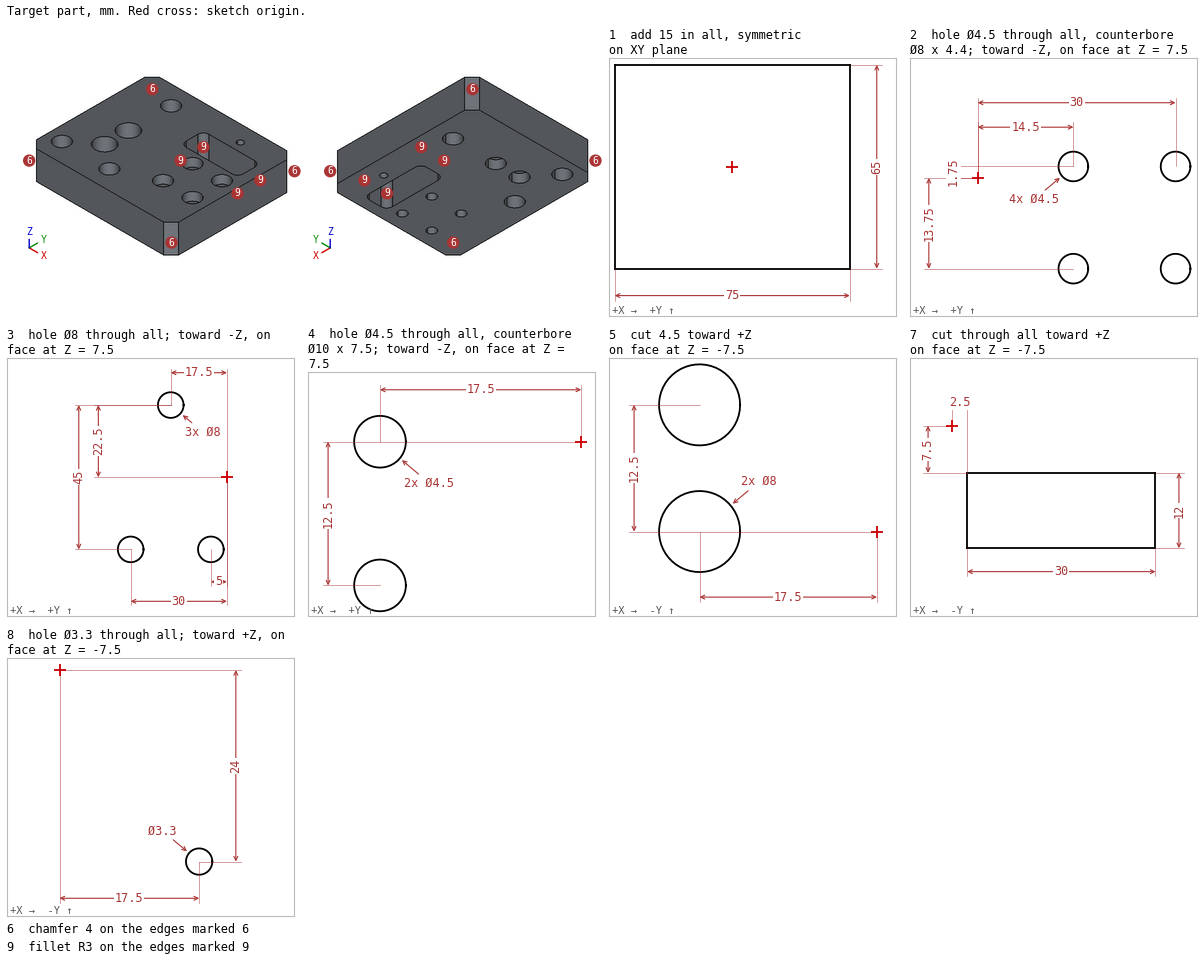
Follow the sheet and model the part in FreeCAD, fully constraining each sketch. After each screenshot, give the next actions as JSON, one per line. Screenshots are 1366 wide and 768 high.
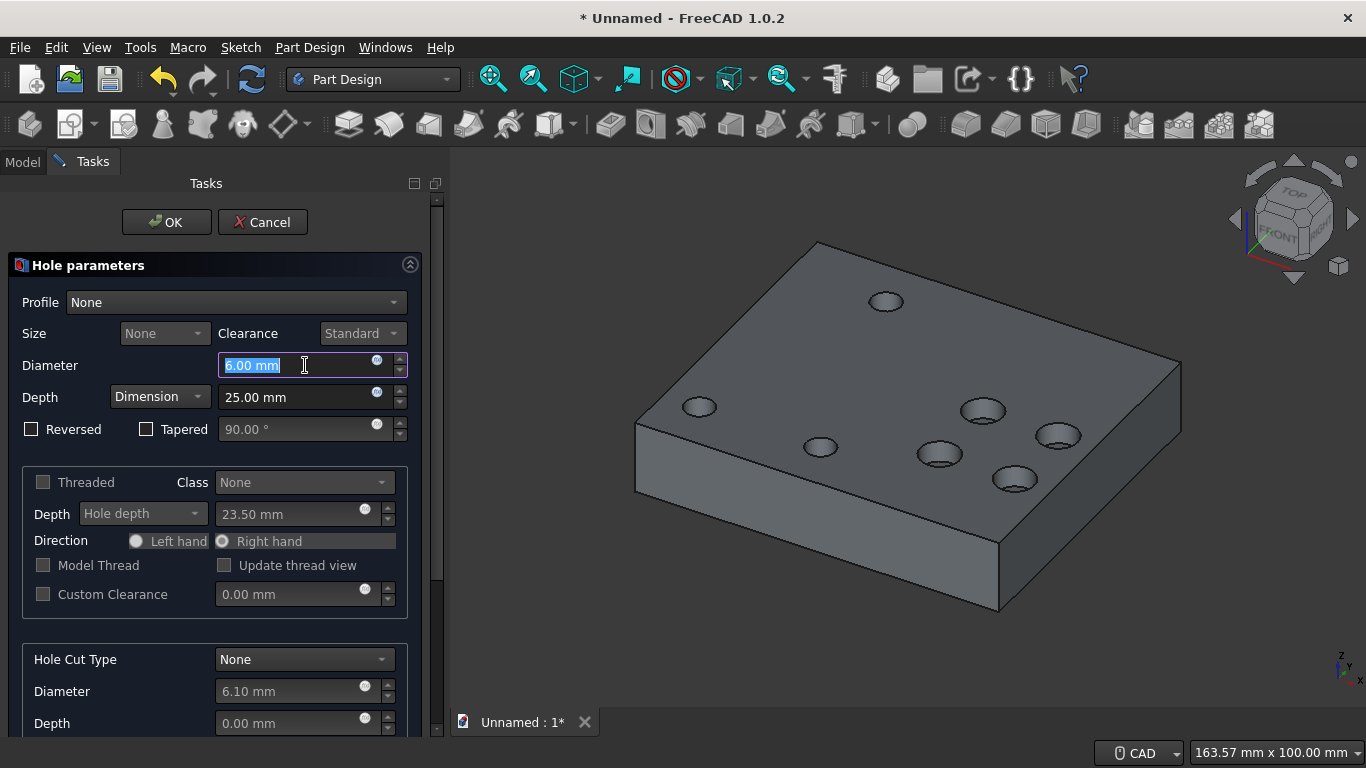
{"action": "type", "text": "8"}
{"action": "key", "text": "Tab"}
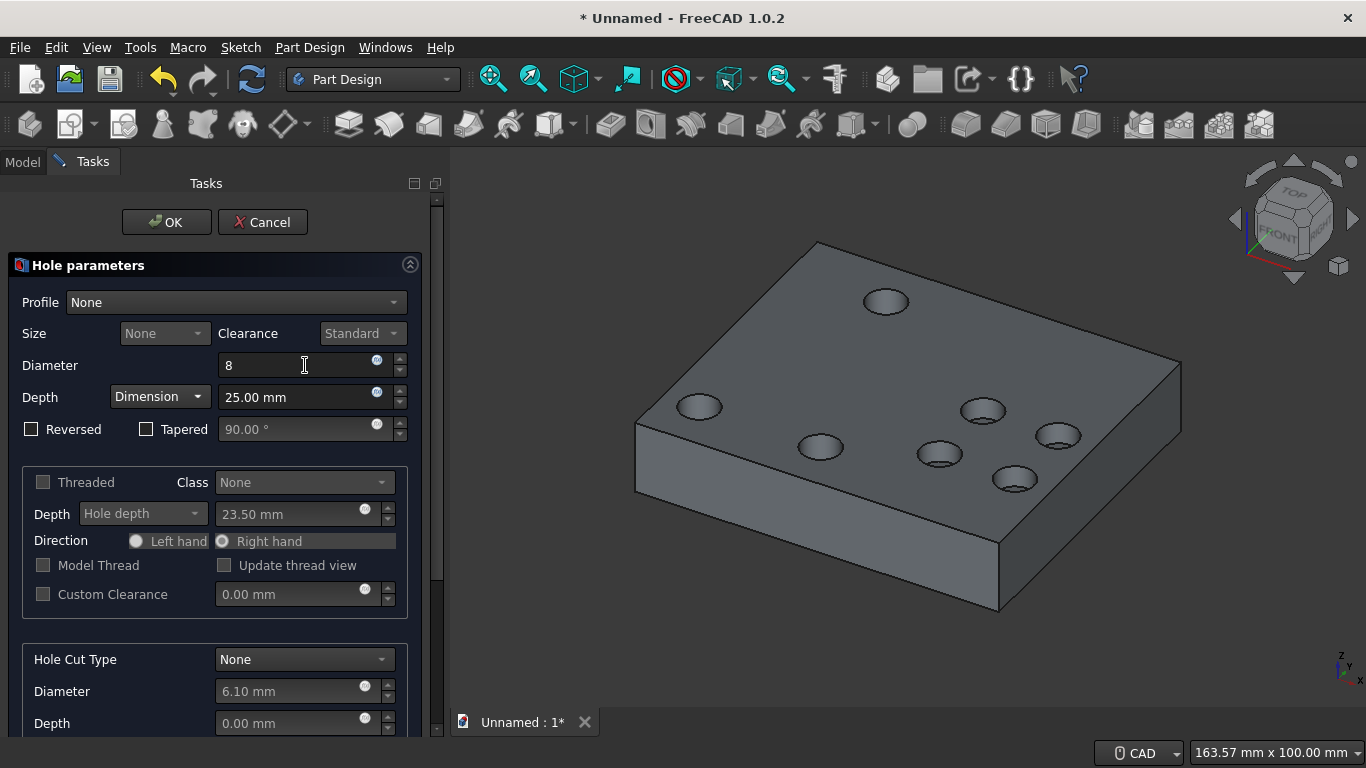
{"action": "left_click", "coordinate": [161, 396]}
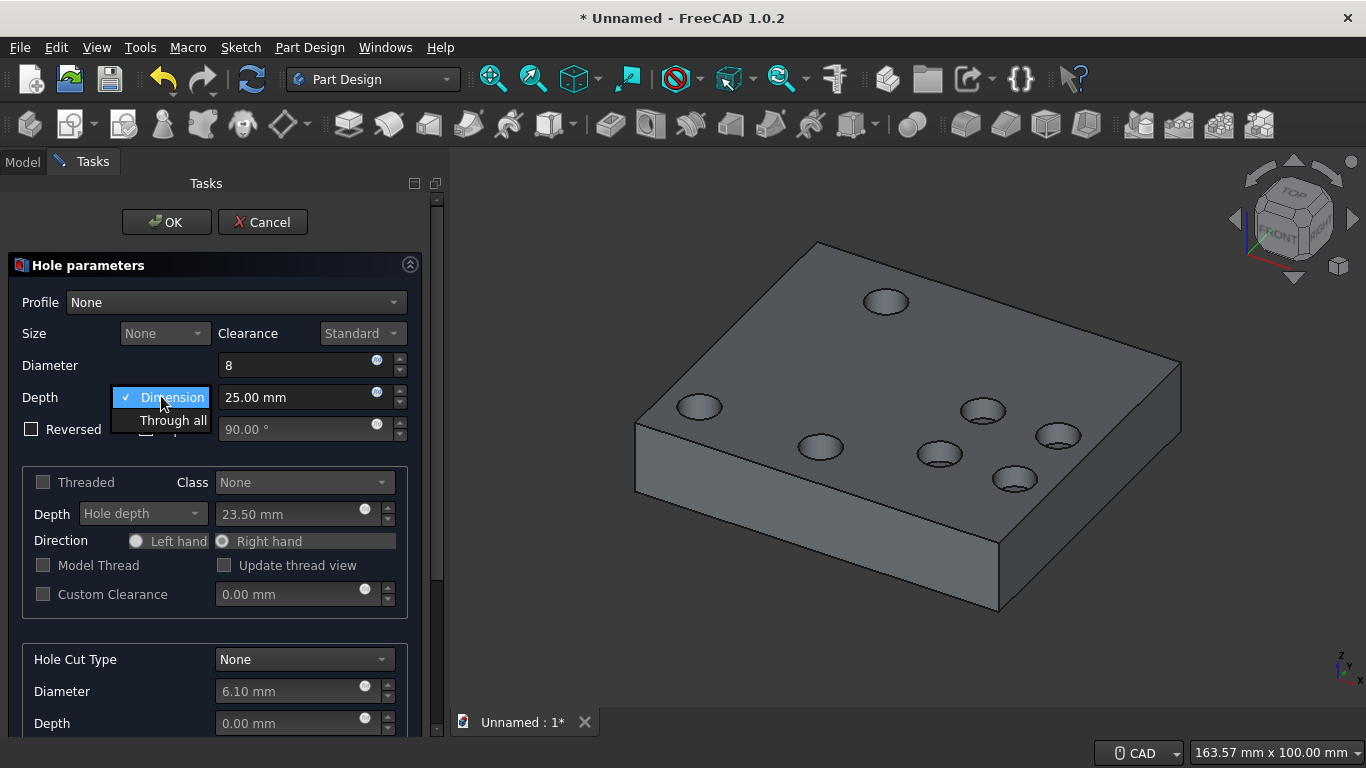
{"action": "left_click", "coordinate": [160, 420]}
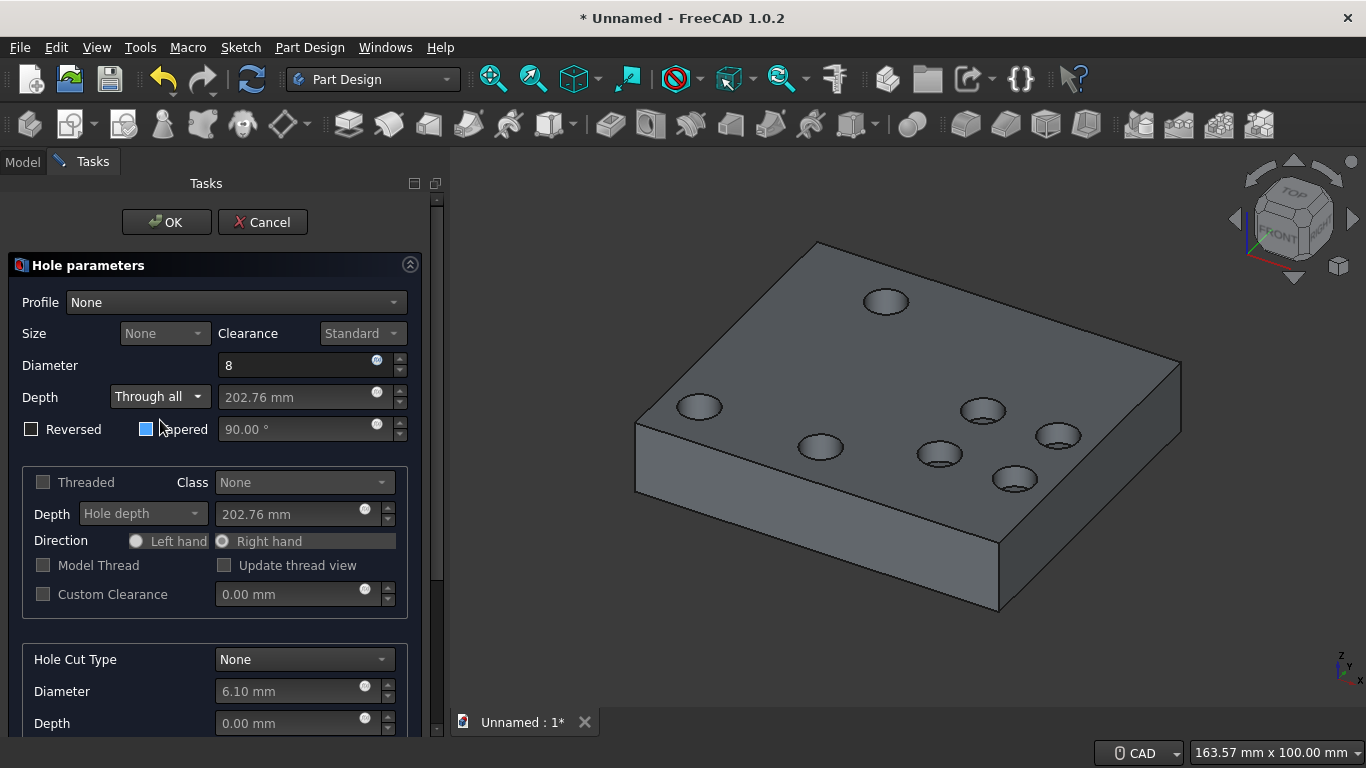
{"action": "left_click", "coordinate": [167, 222]}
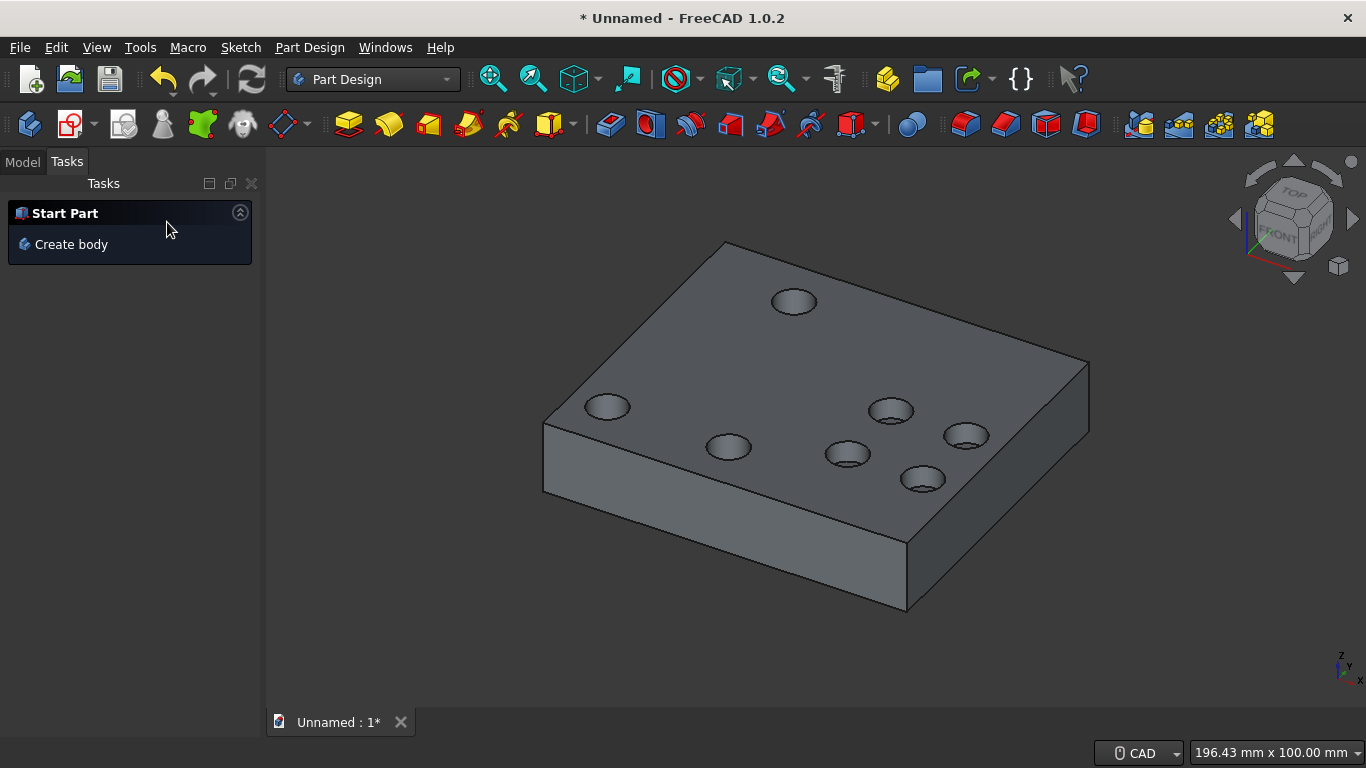
{"action": "left_click", "coordinate": [764, 374]}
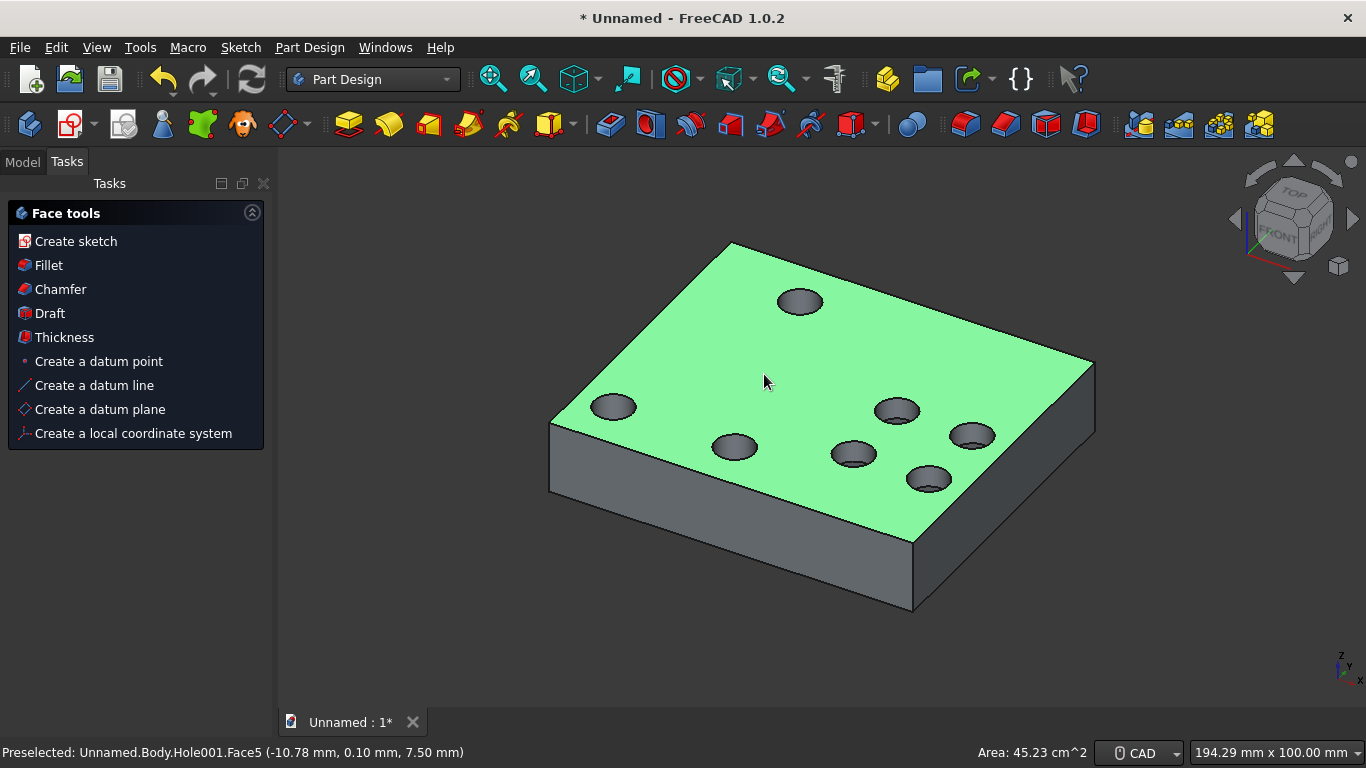
{"action": "left_click", "coordinate": [70, 124]}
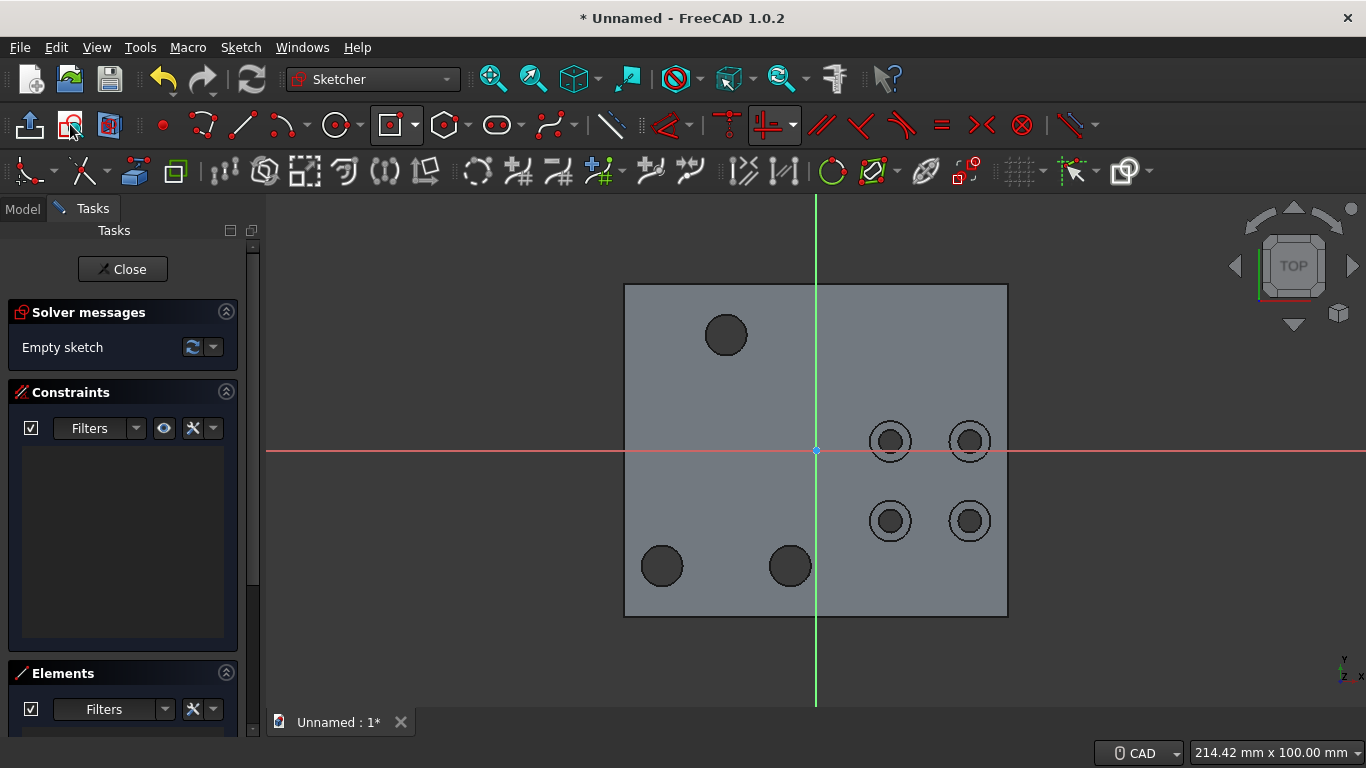
{"action": "scroll", "coordinate": [771, 493], "scroll_direction": "up", "scroll_amount": 7}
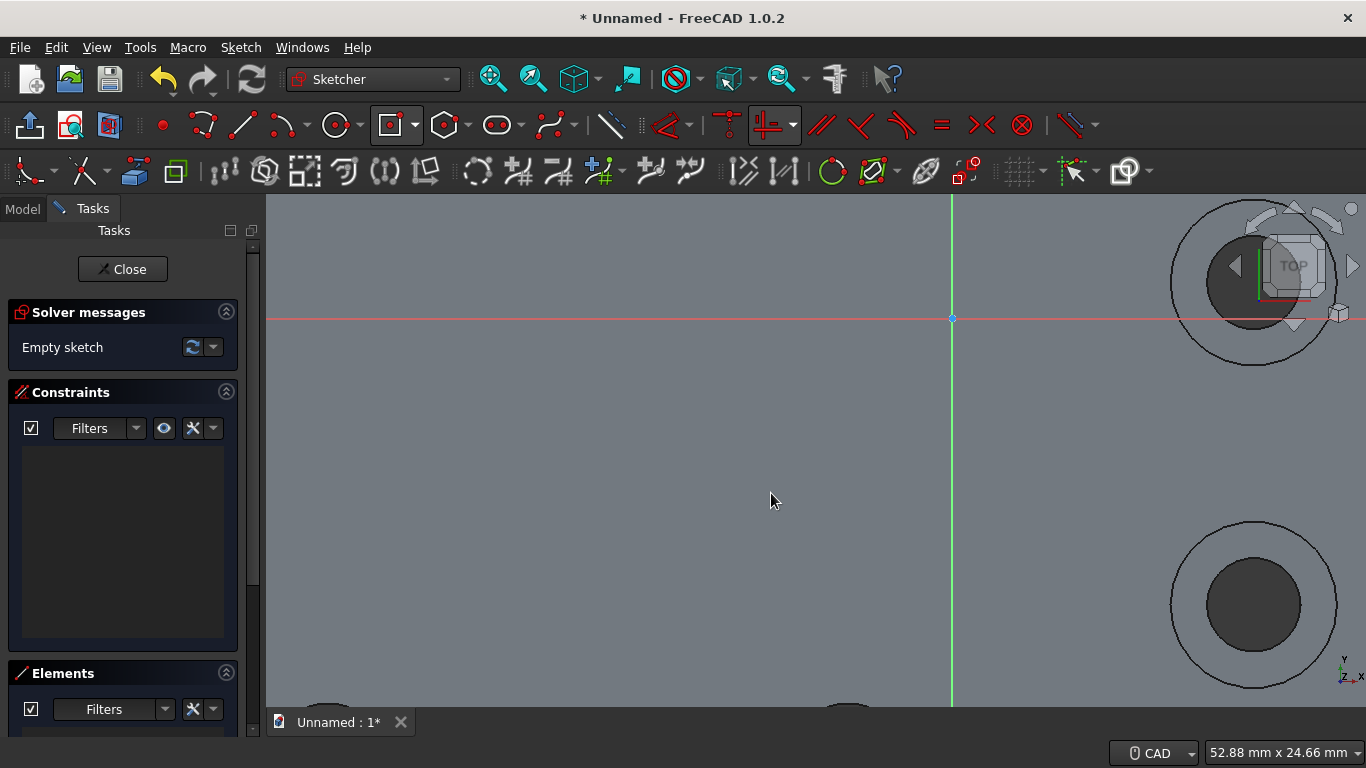
{"action": "left_click", "coordinate": [336, 126]}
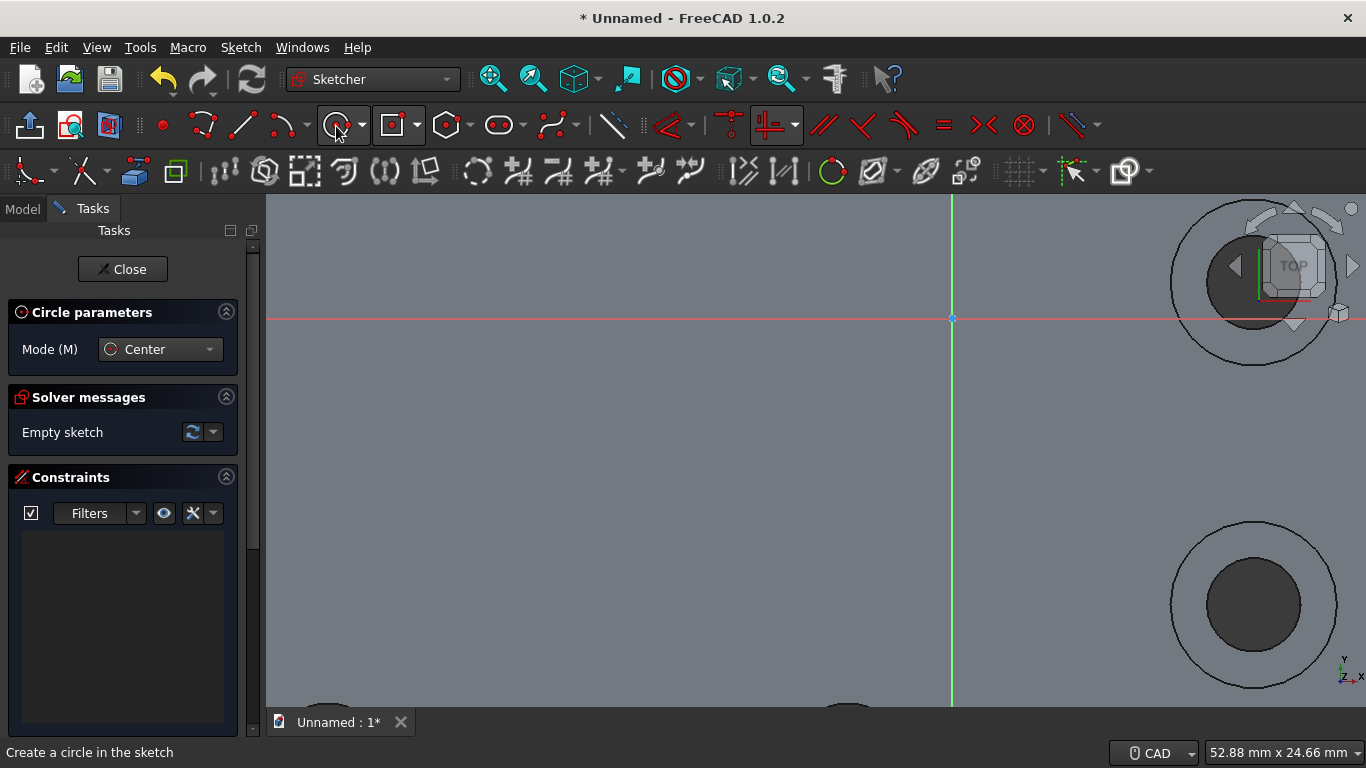
{"action": "left_click", "coordinate": [588, 319]}
{"action": "mouse_move", "coordinate": [621, 286]}